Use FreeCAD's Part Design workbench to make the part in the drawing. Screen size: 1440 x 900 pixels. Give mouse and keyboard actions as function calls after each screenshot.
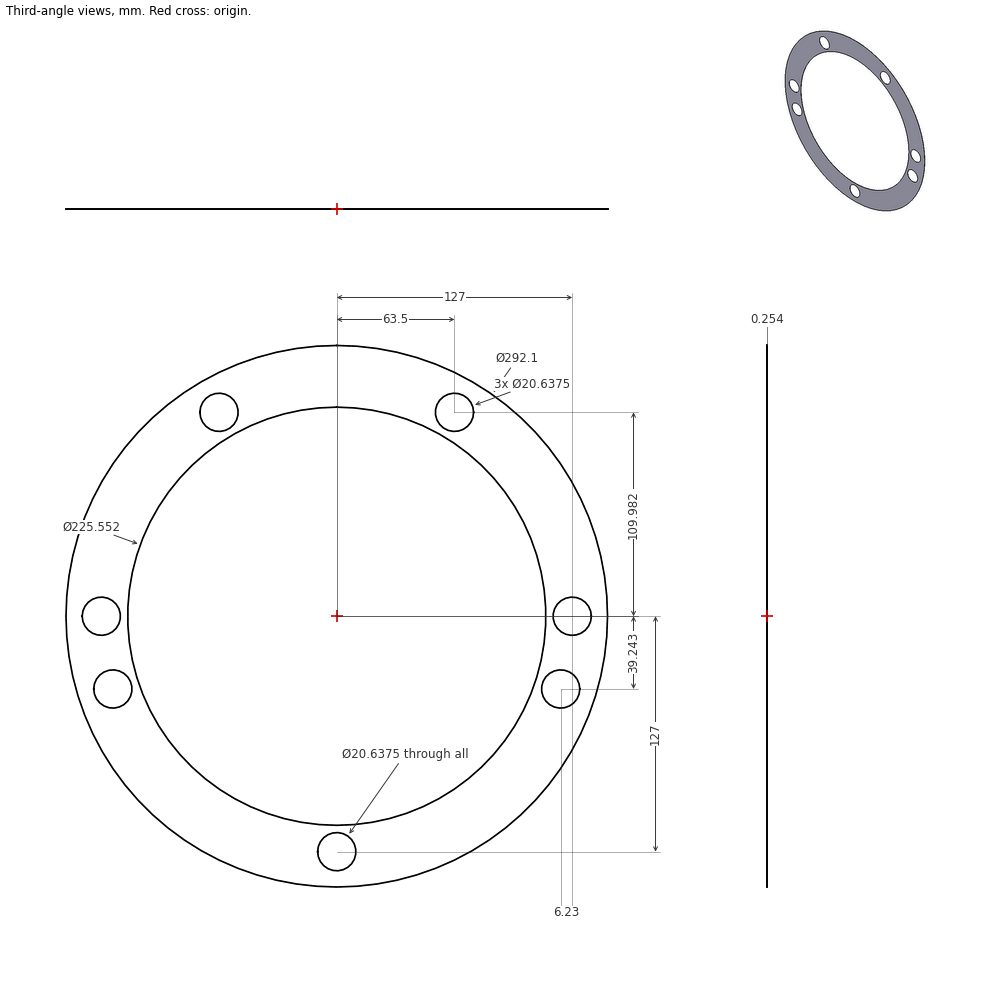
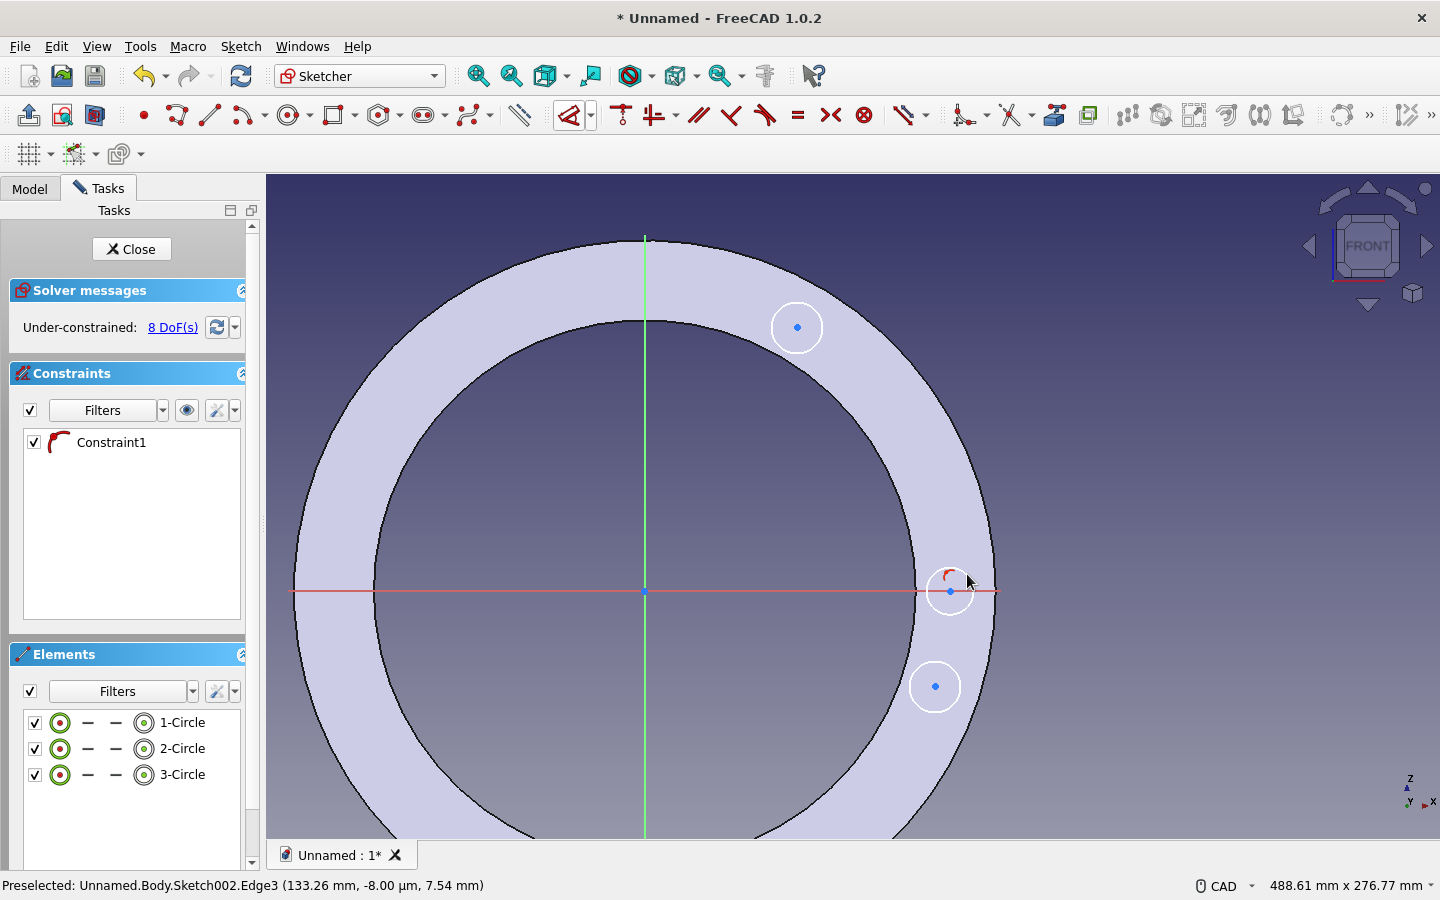
click(815, 310)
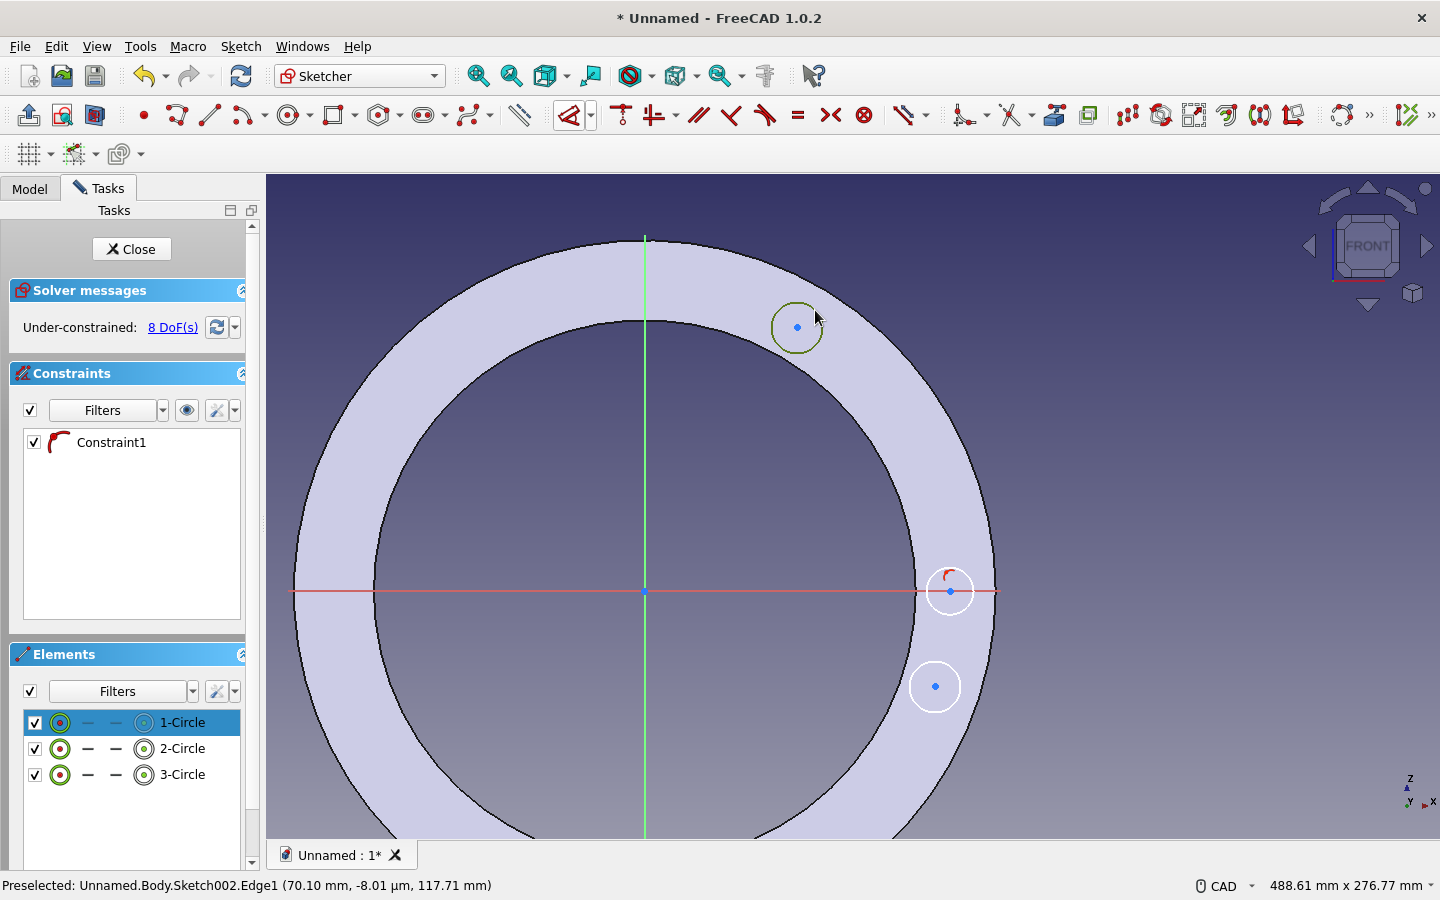
click(953, 669)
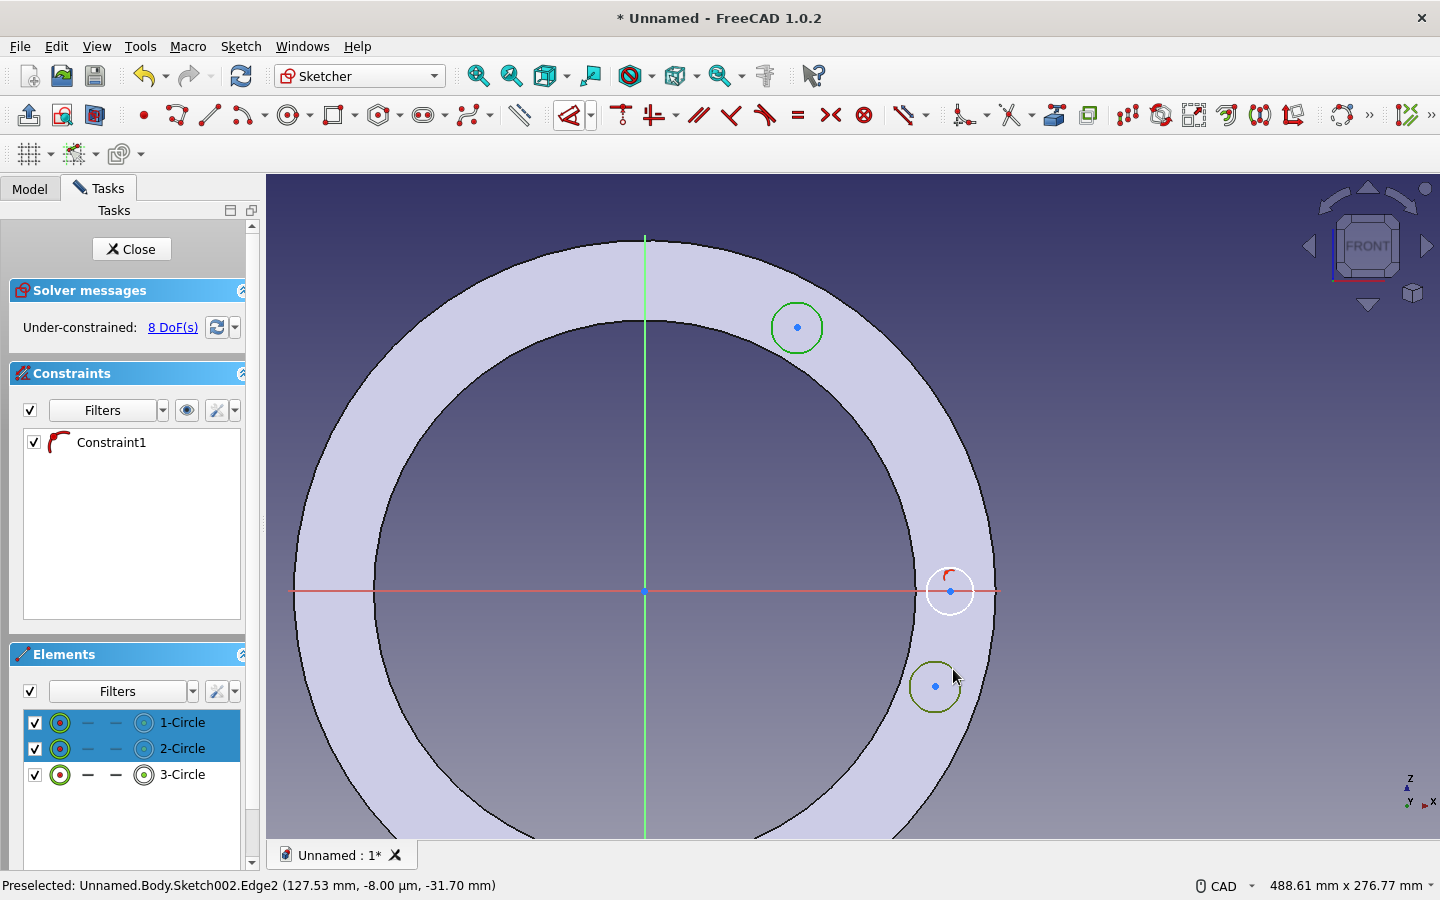
click(967, 575)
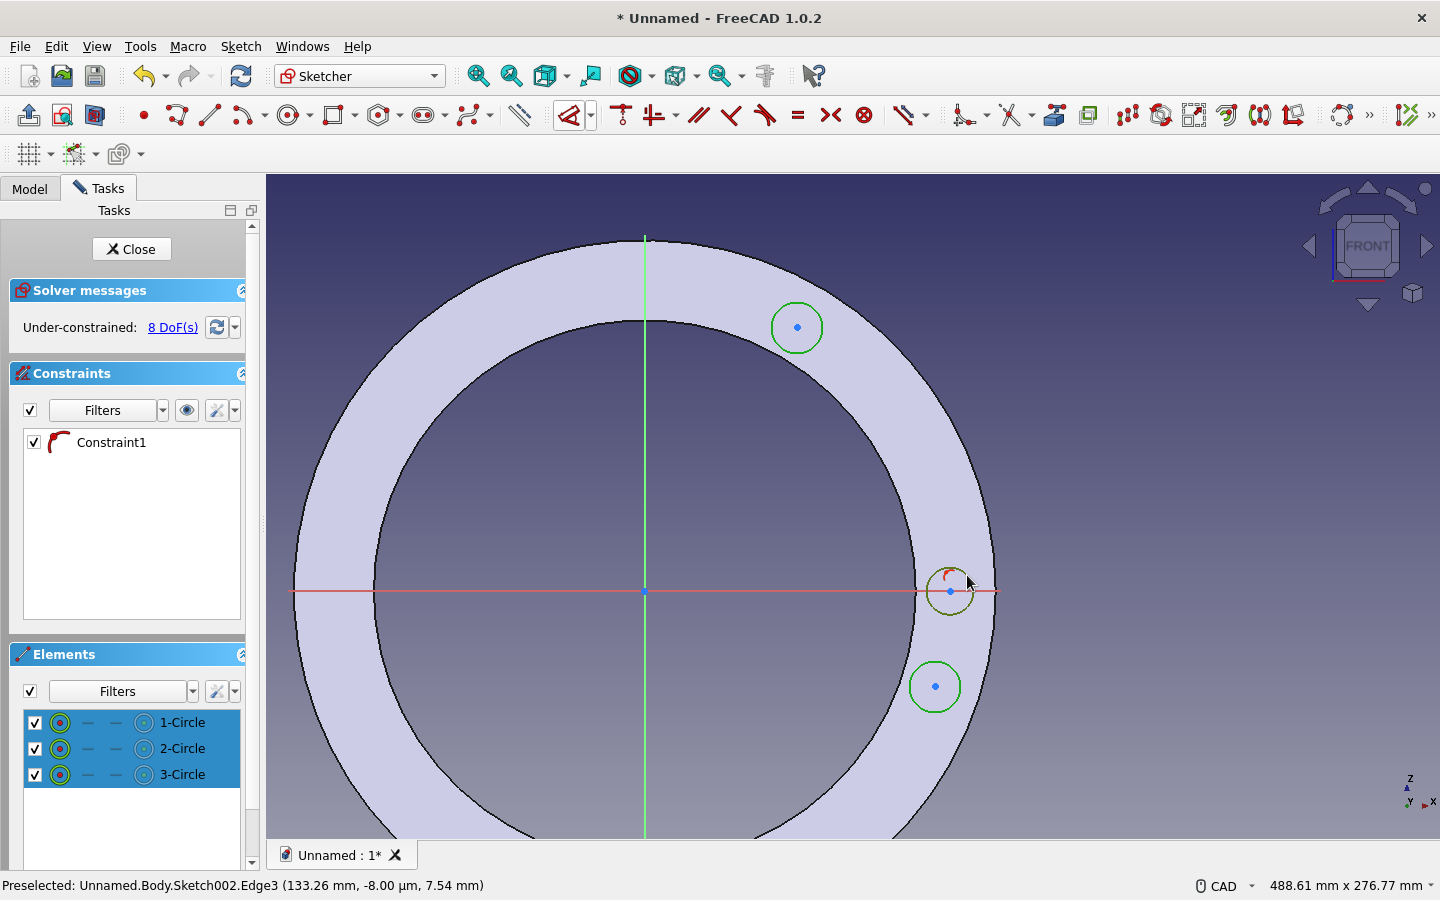
click(798, 116)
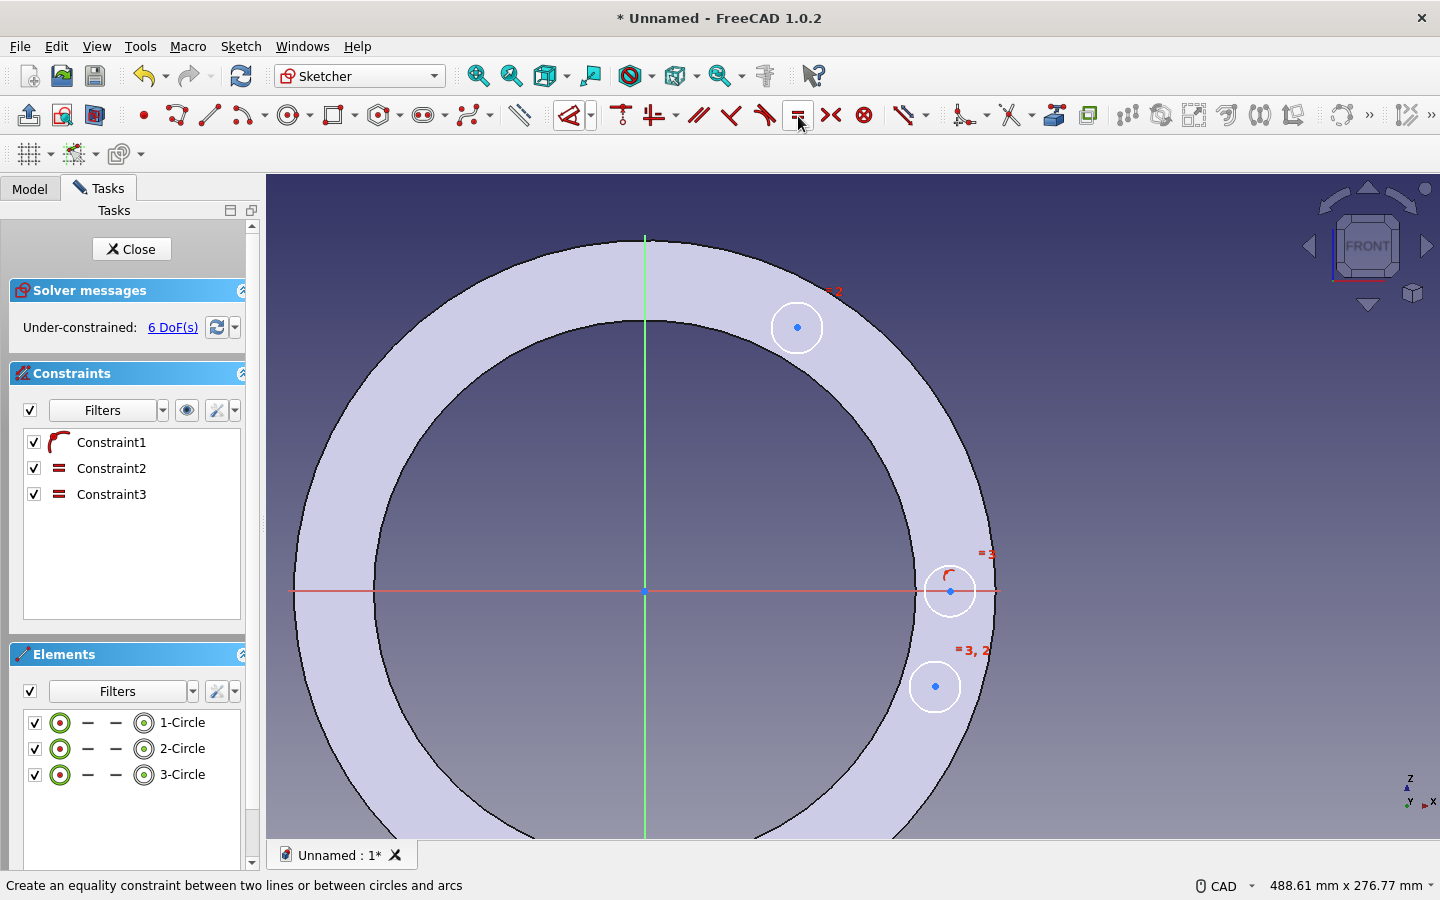
click(815, 310)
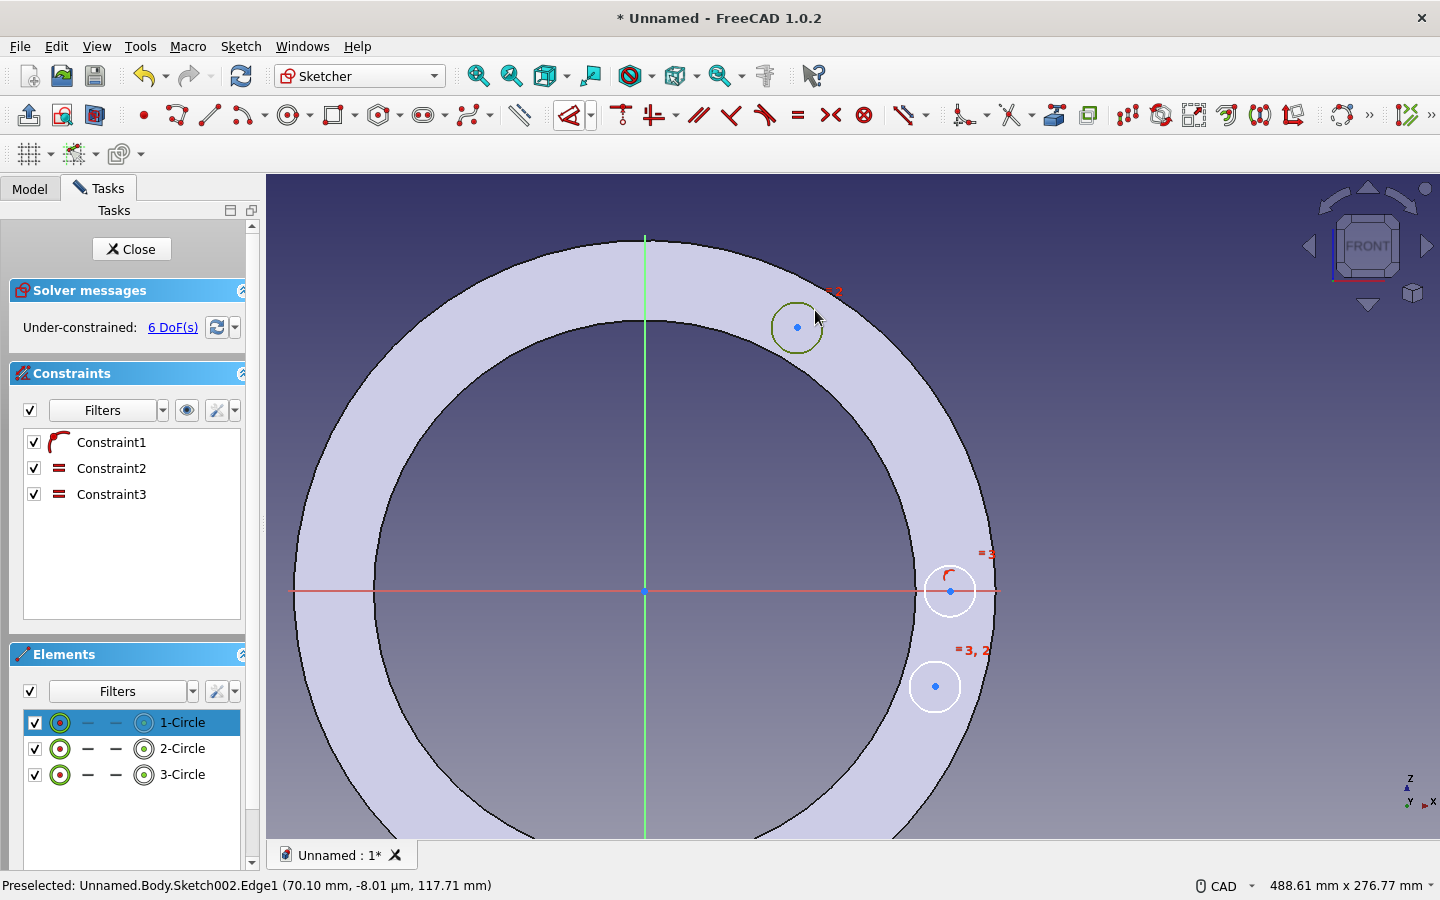
click(590, 116)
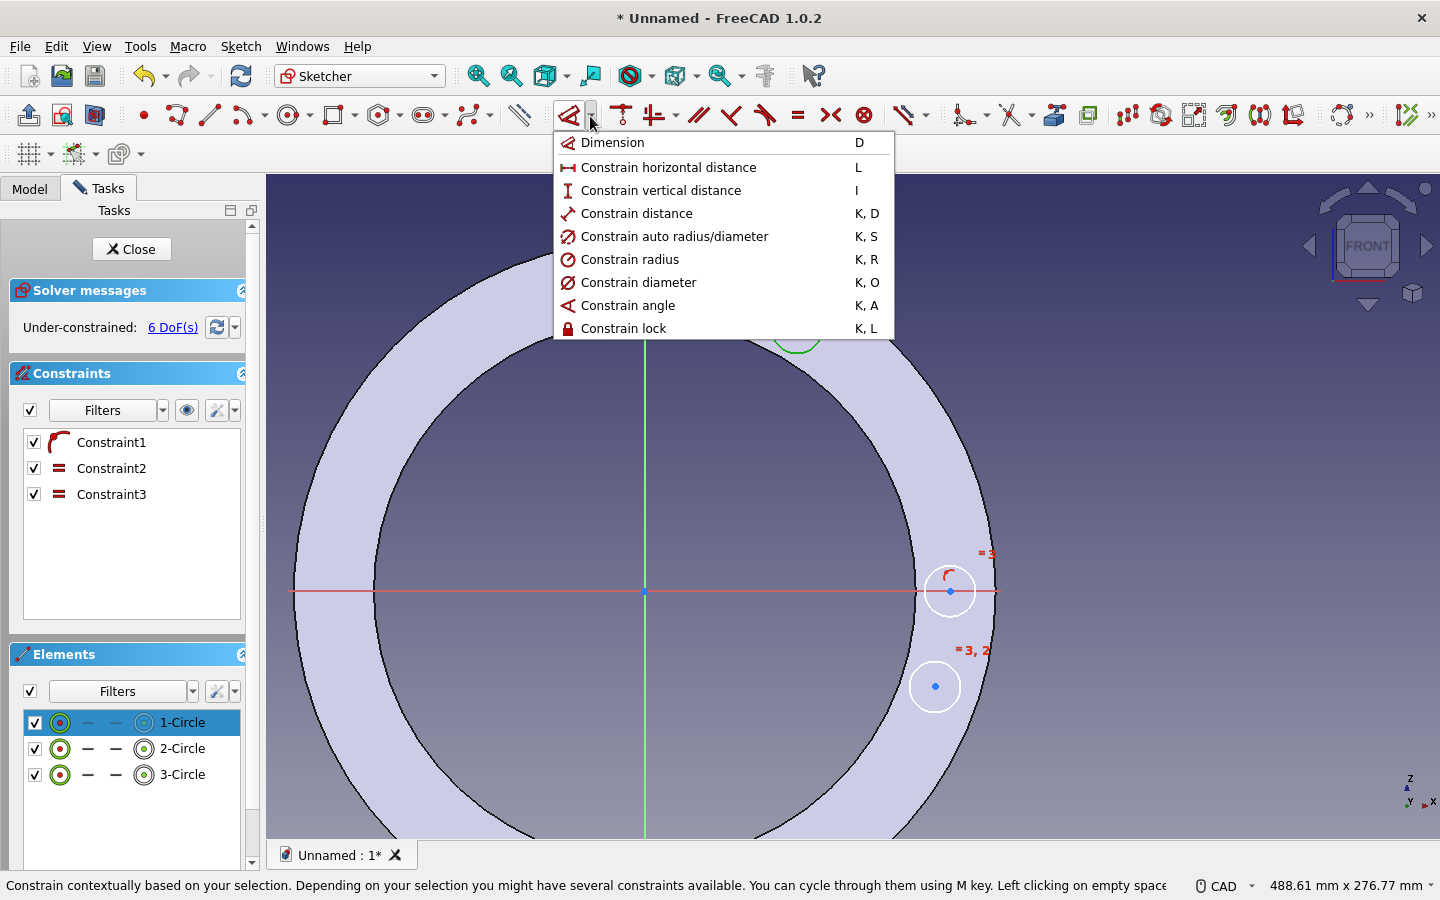
click(724, 282)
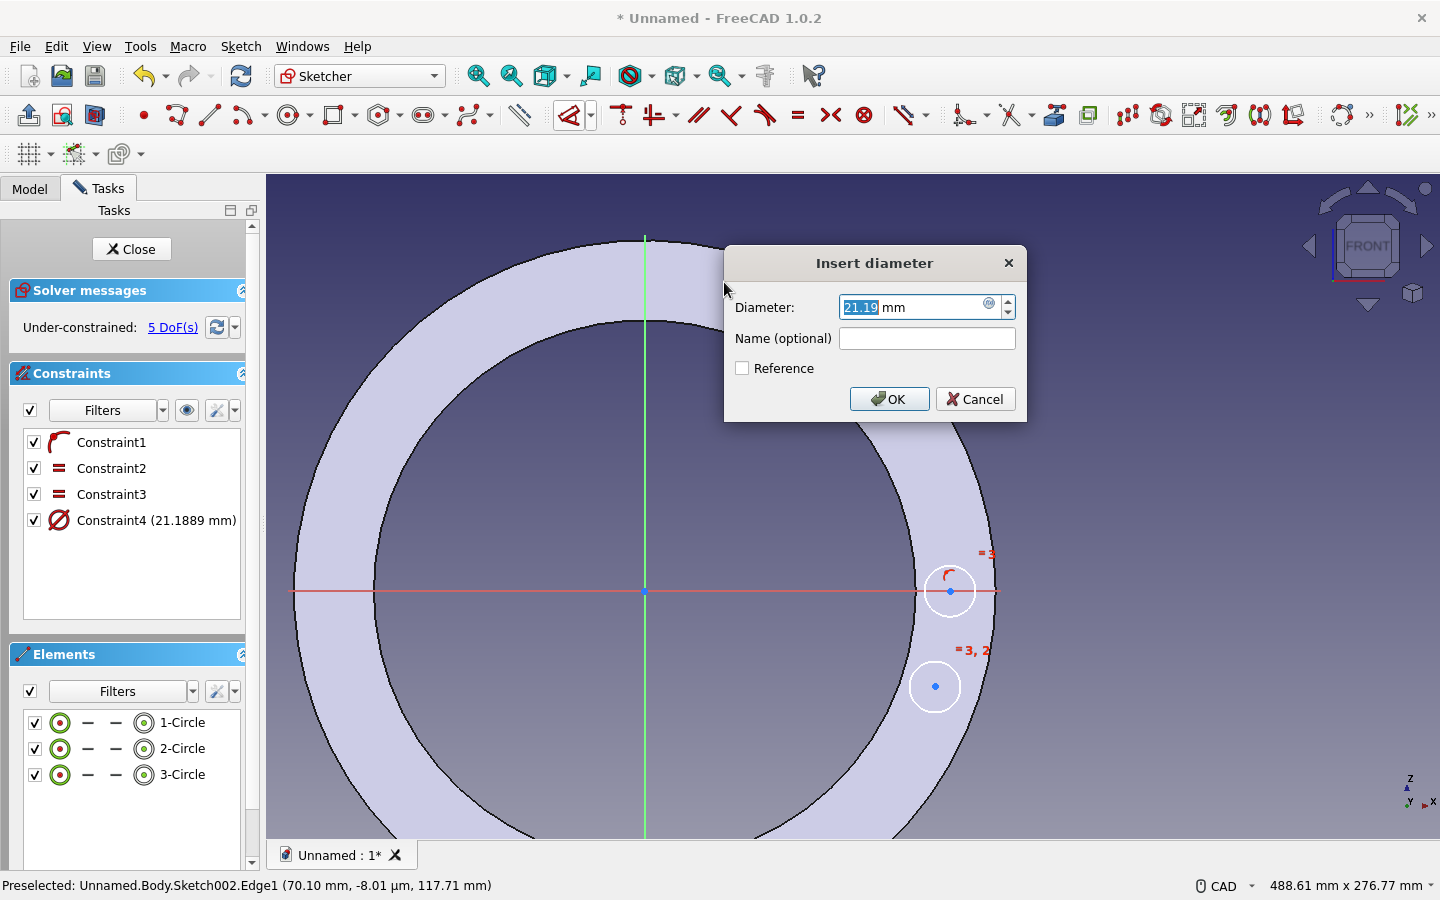
text(20.6375)
key(Return)